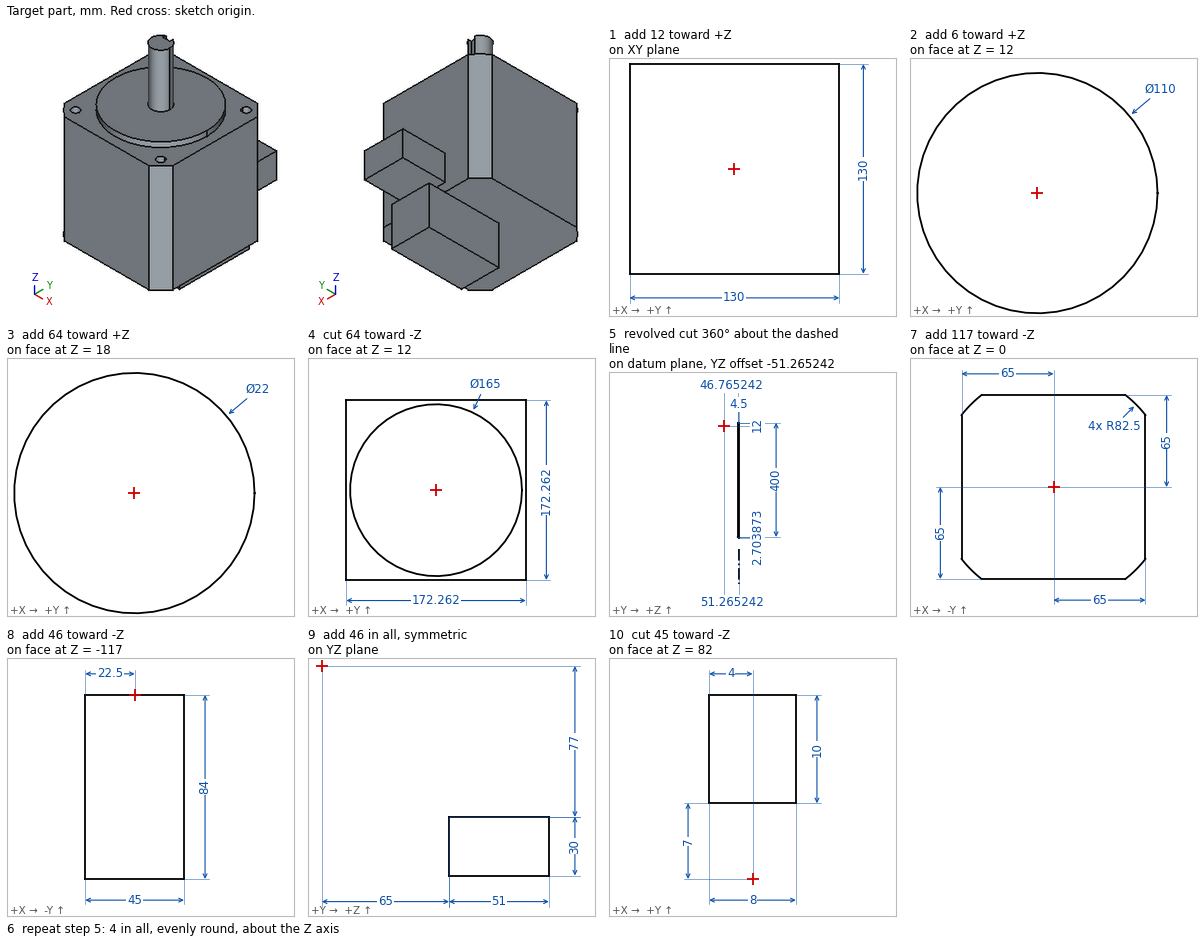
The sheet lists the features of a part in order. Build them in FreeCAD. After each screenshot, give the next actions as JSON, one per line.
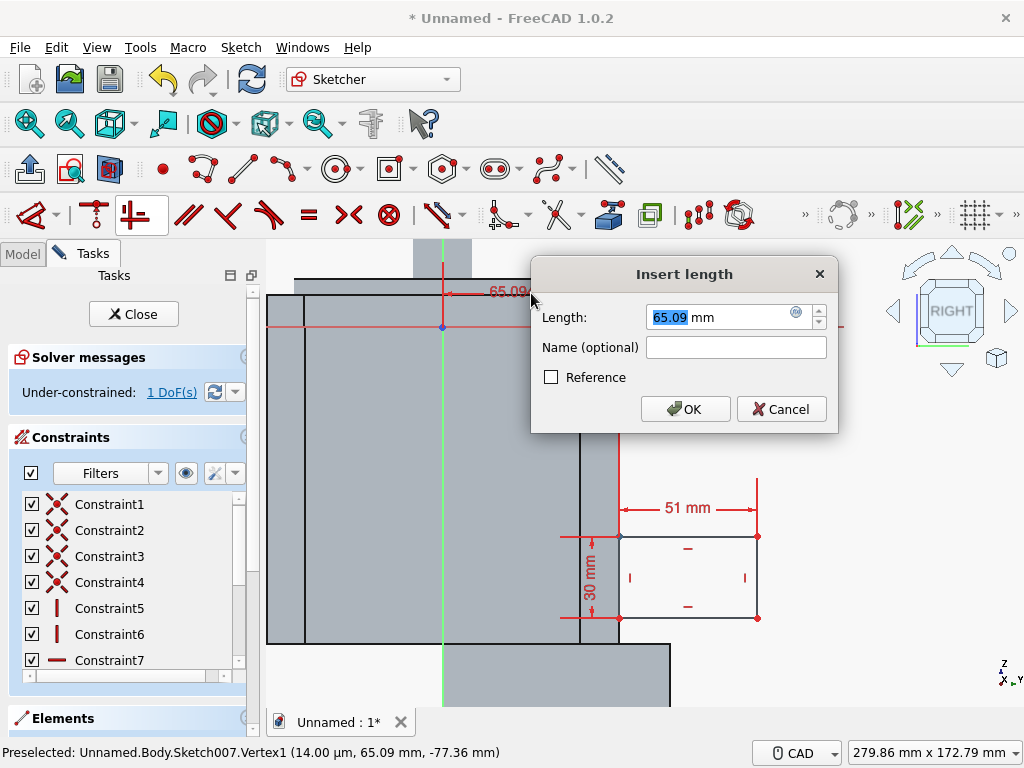
{"action": "type", "text": "65"}
{"action": "key", "text": "Return"}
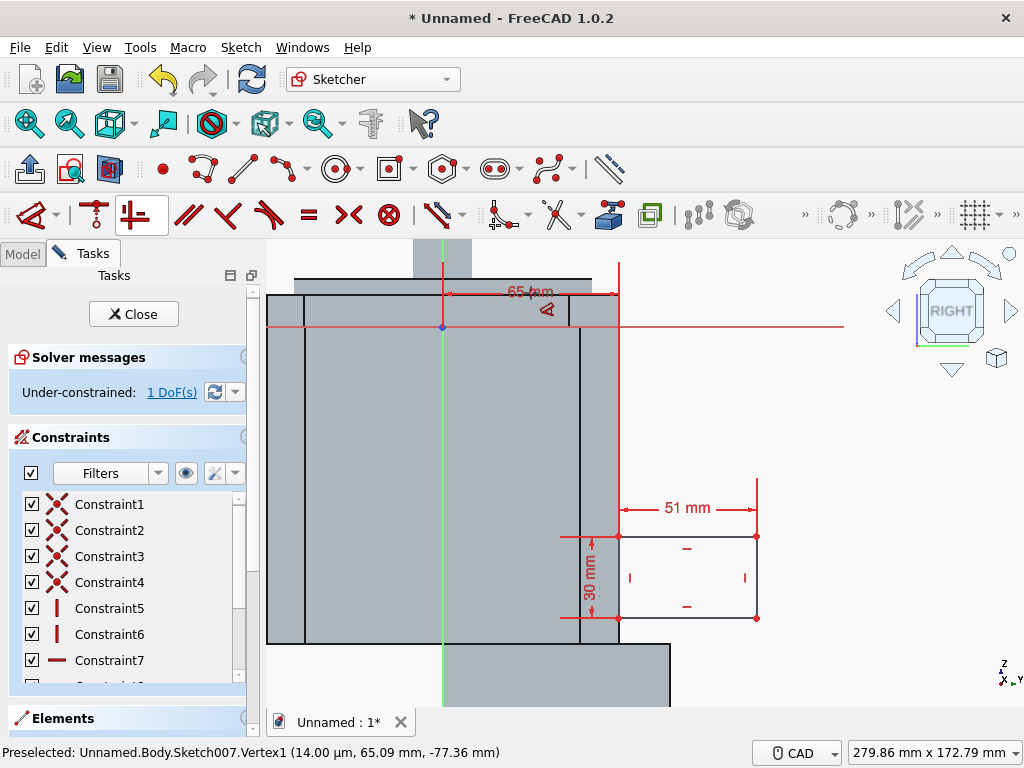
{"action": "left_click", "coordinate": [619, 537]}
{"action": "left_click", "coordinate": [409, 432]}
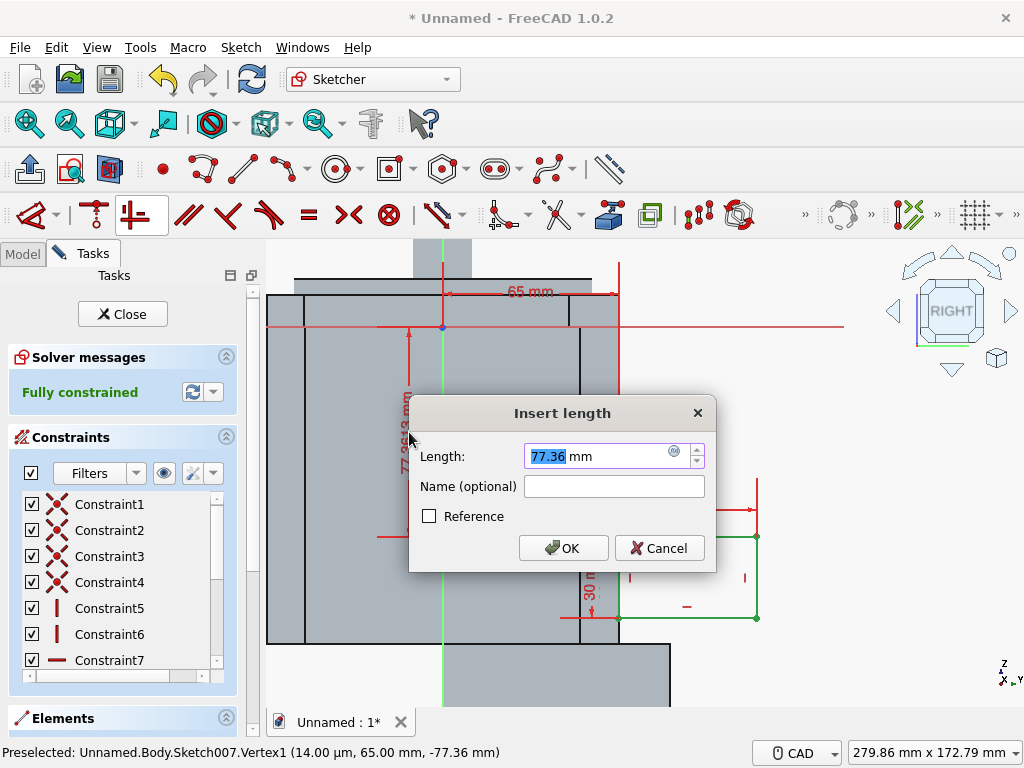
{"action": "type", "text": "77"}
{"action": "key", "text": "Return"}
{"action": "key", "text": "Escape"}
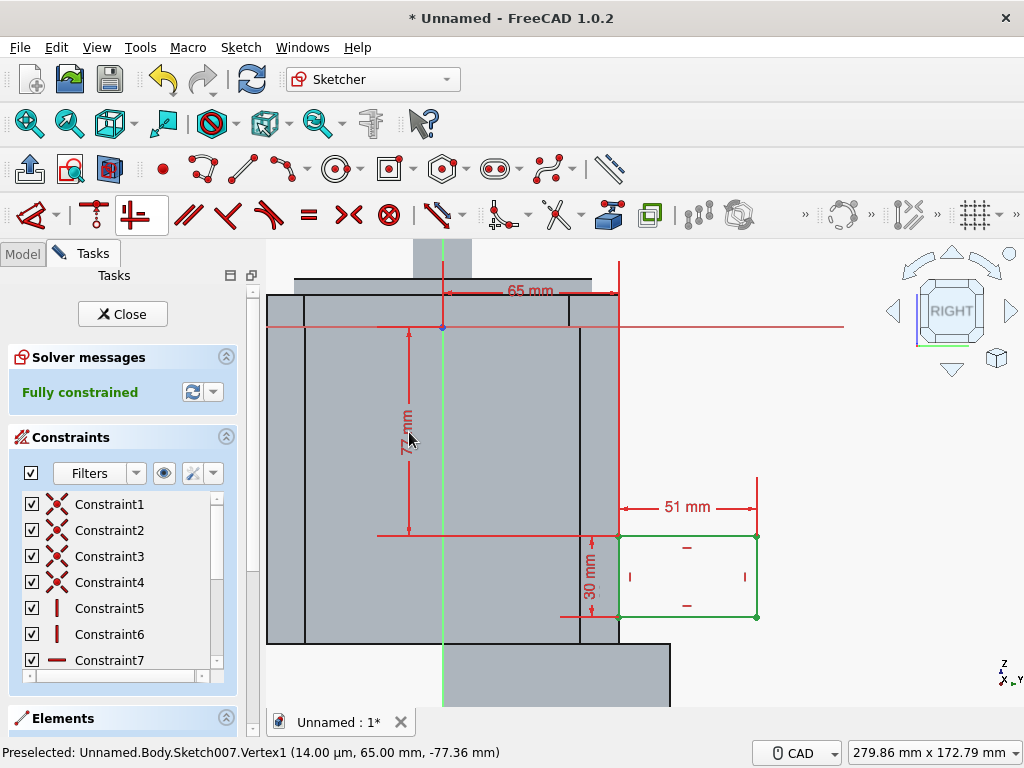
{"action": "left_click", "coordinate": [123, 314]}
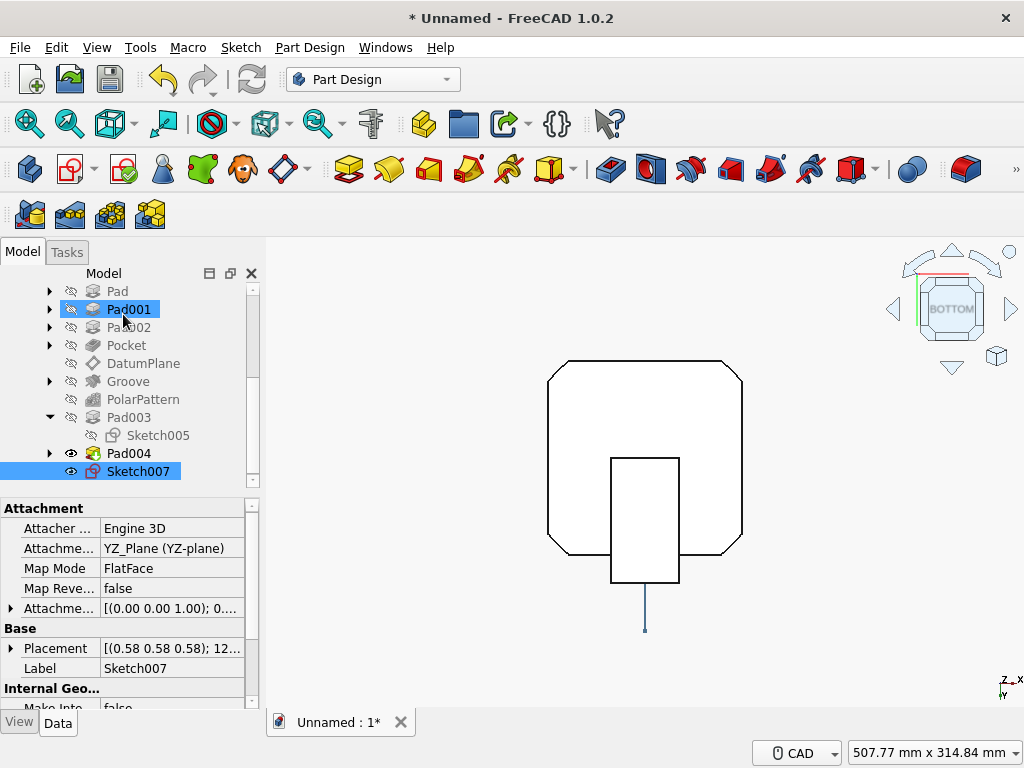
{"action": "left_click", "coordinate": [350, 170]}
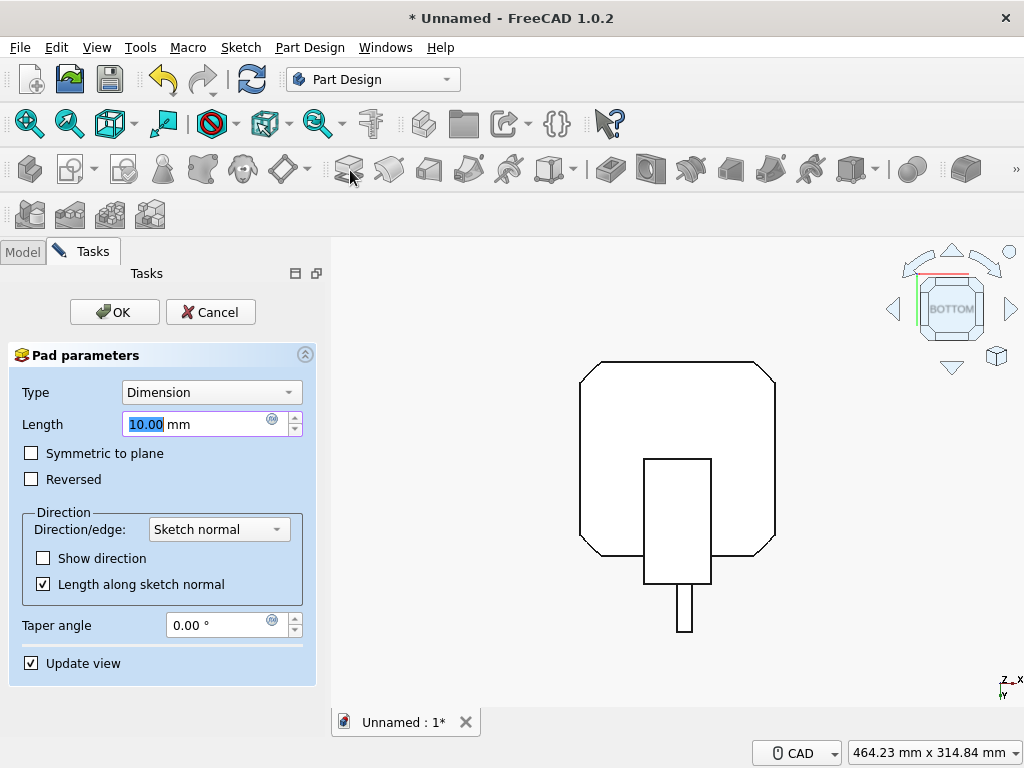
{"action": "type", "text": "46"}
{"action": "key", "text": "Tab"}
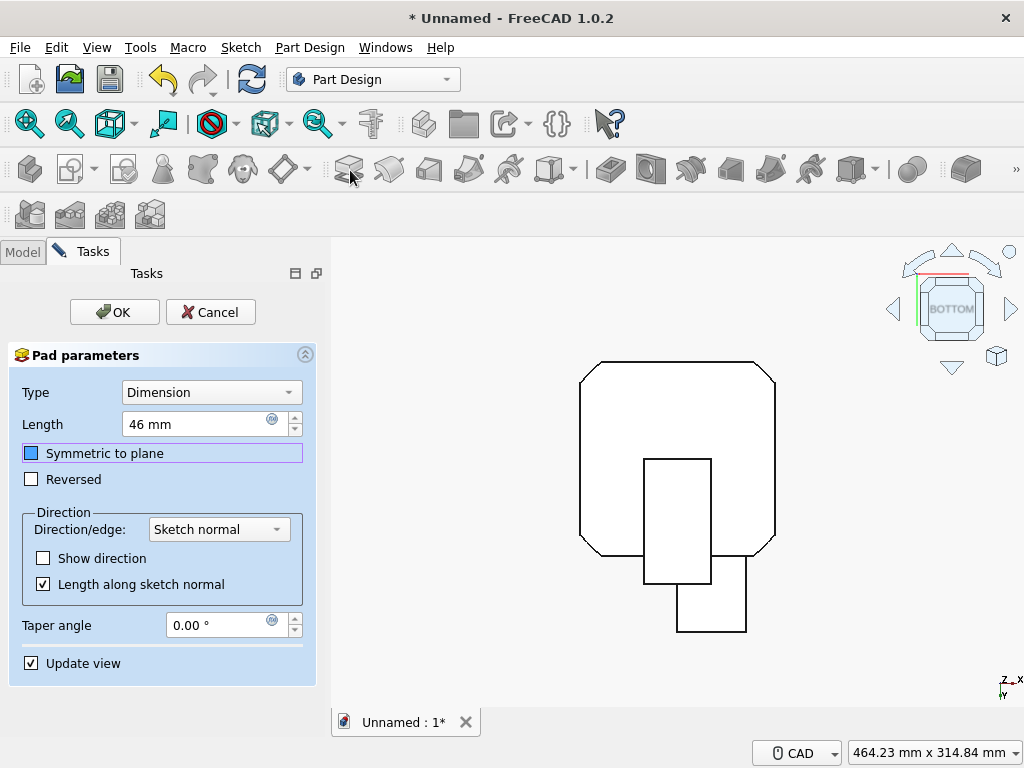
{"action": "left_click", "coordinate": [30, 453]}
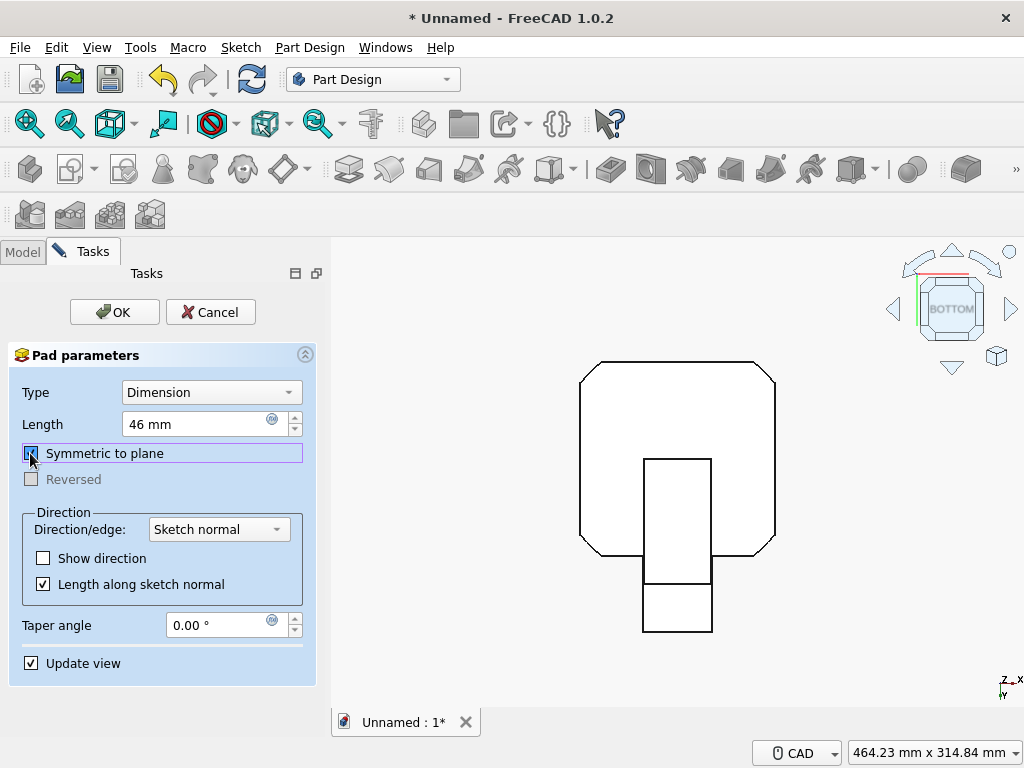
{"action": "left_click", "coordinate": [115, 312]}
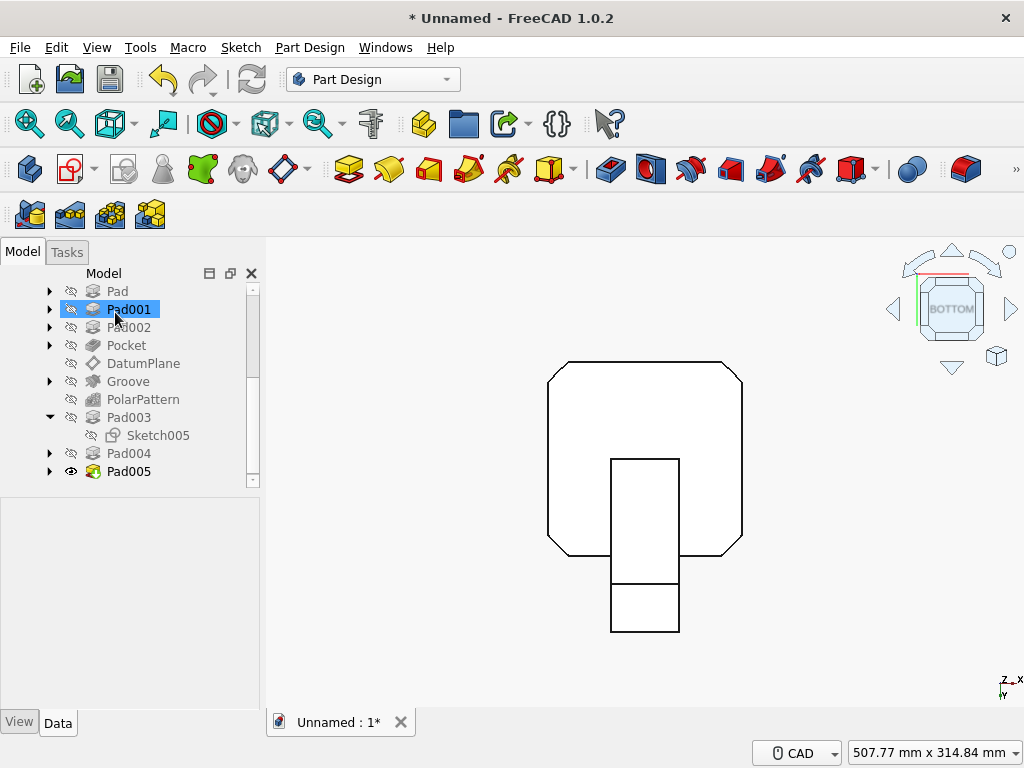
{"action": "key", "text": "0"}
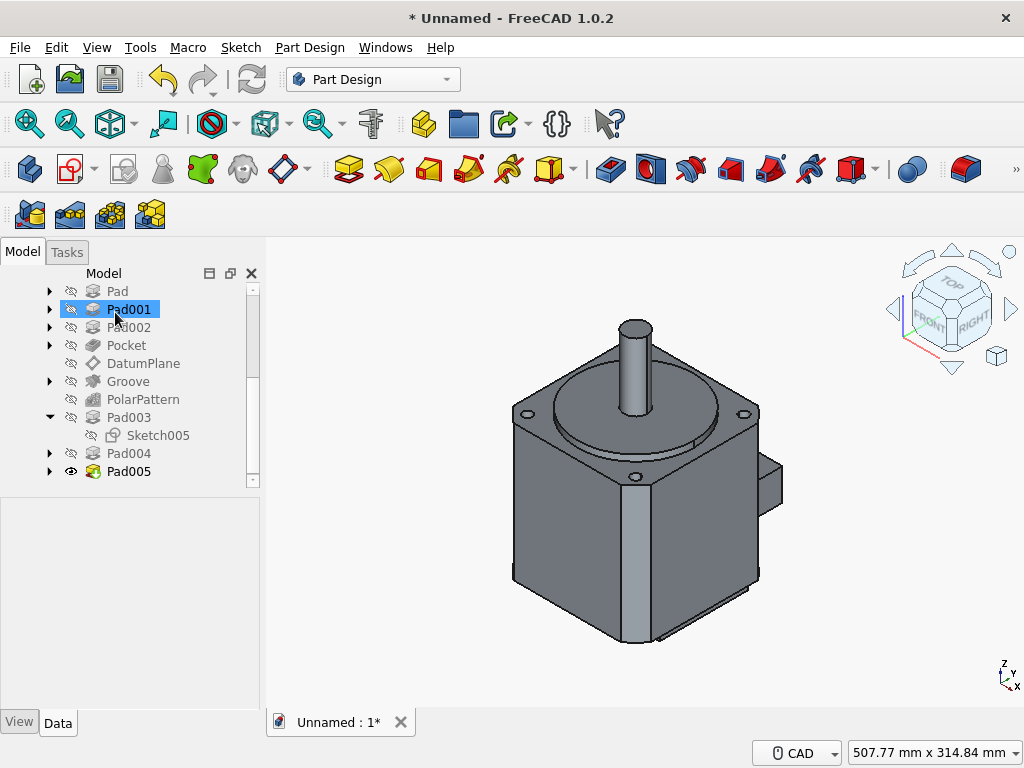
{"action": "left_click", "coordinate": [30, 124]}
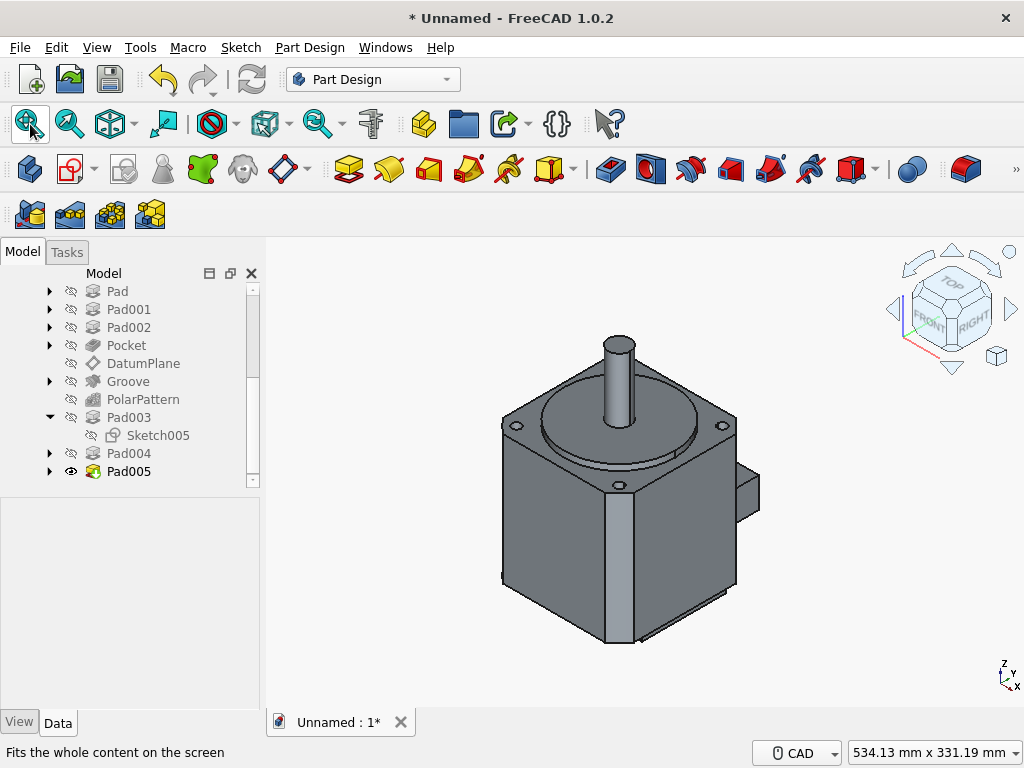
{"action": "left_click", "coordinate": [619, 344]}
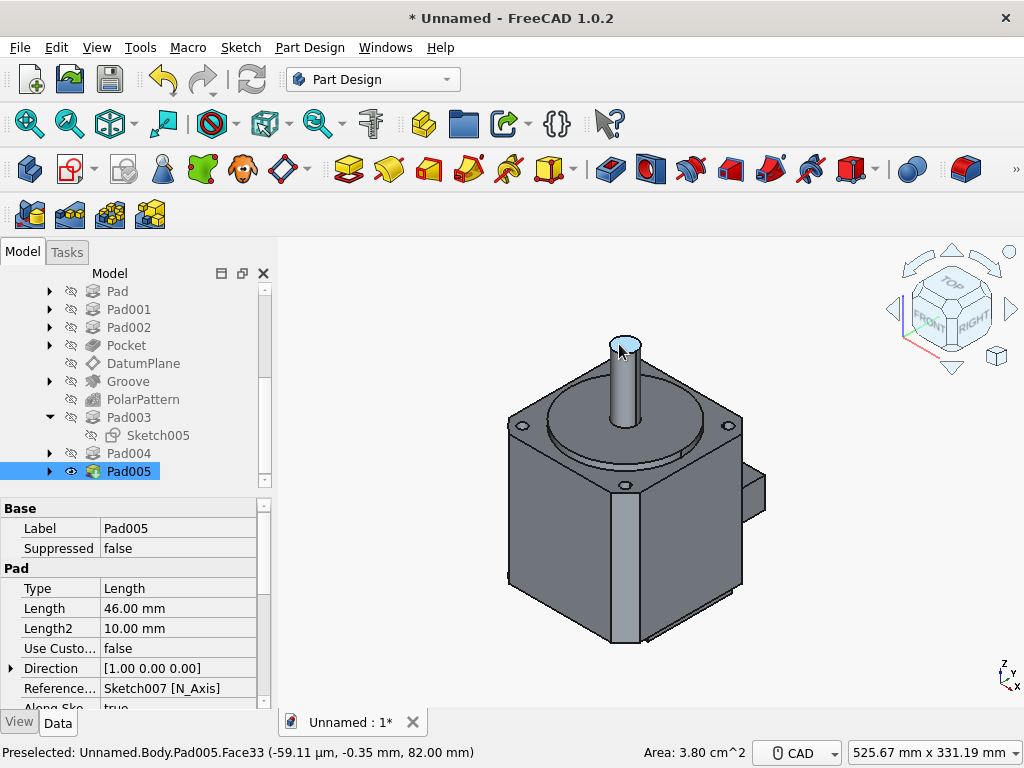
{"action": "left_click", "coordinate": [70, 170]}